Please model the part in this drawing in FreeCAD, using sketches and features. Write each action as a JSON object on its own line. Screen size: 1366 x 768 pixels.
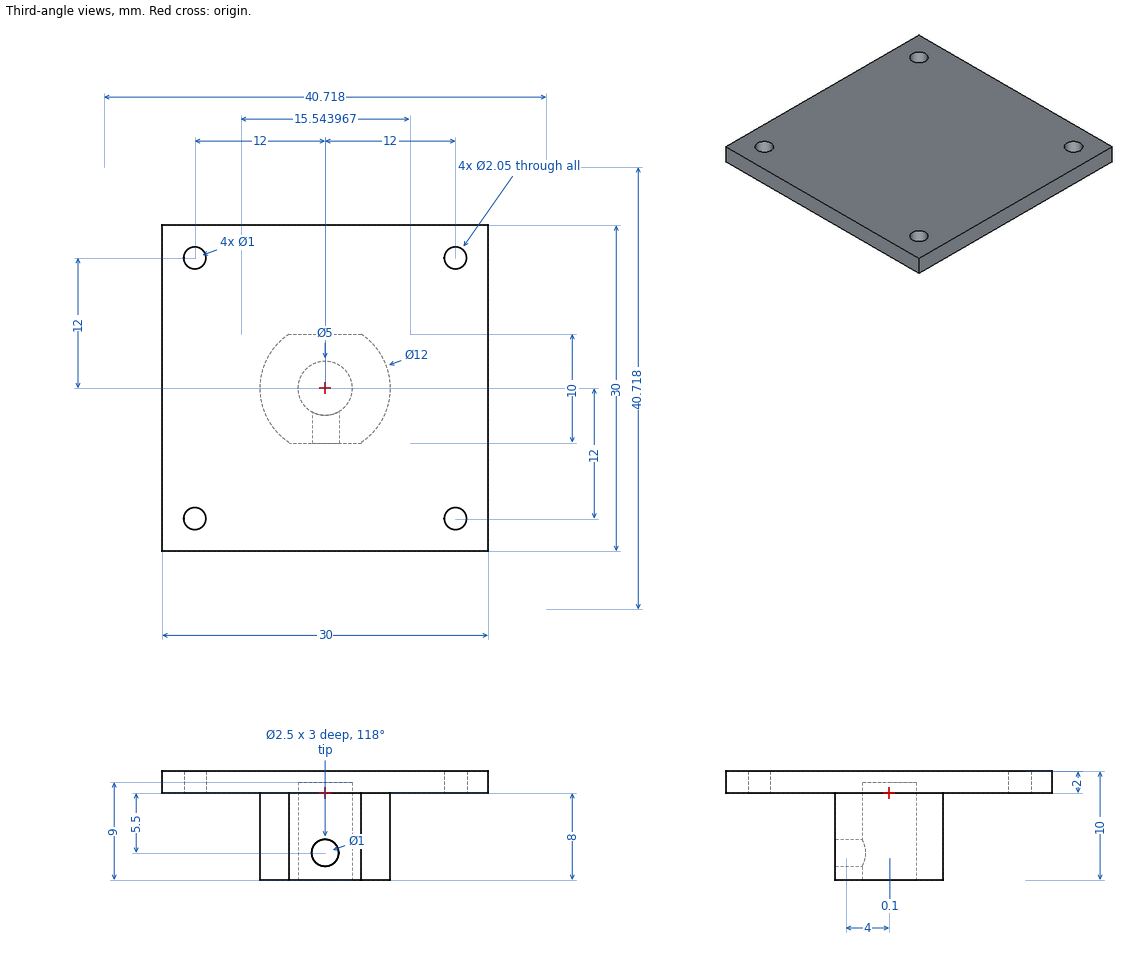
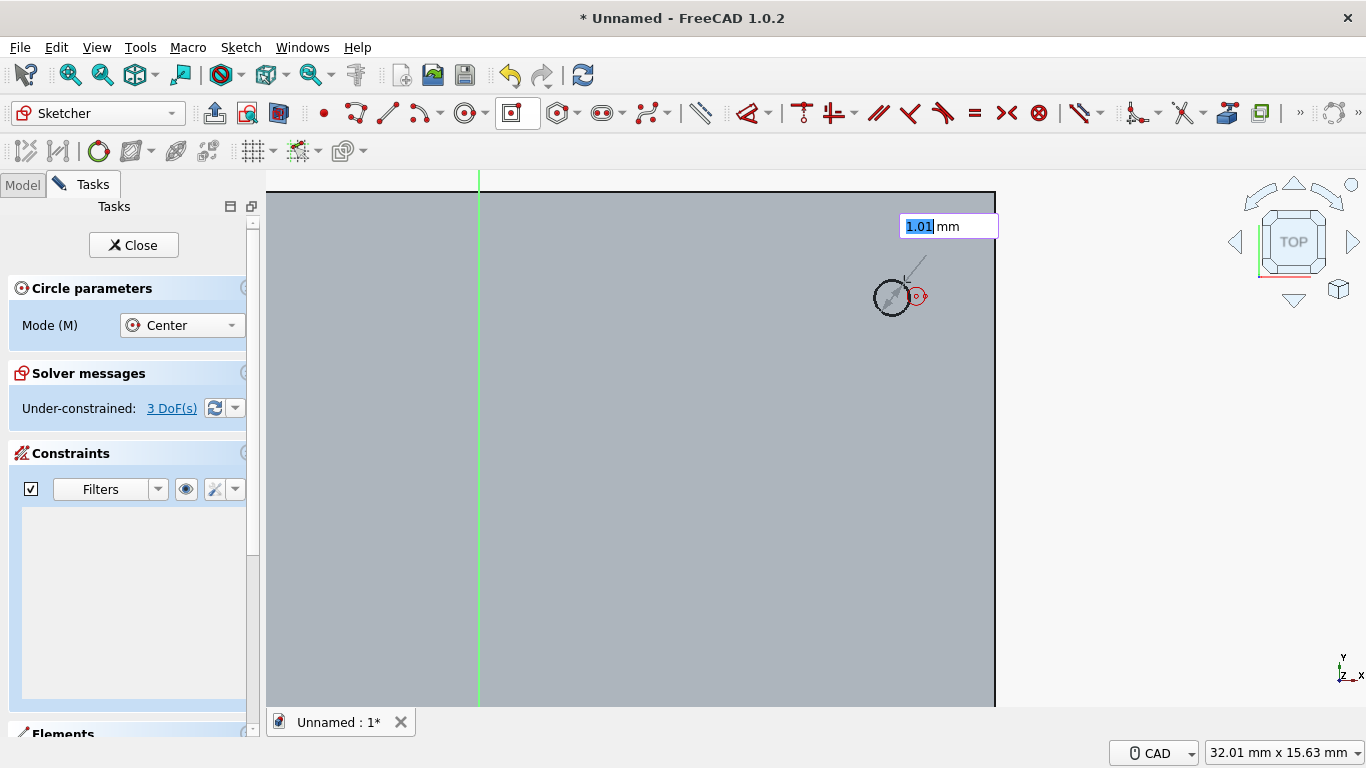
{"action": "left_click", "coordinate": [904, 282]}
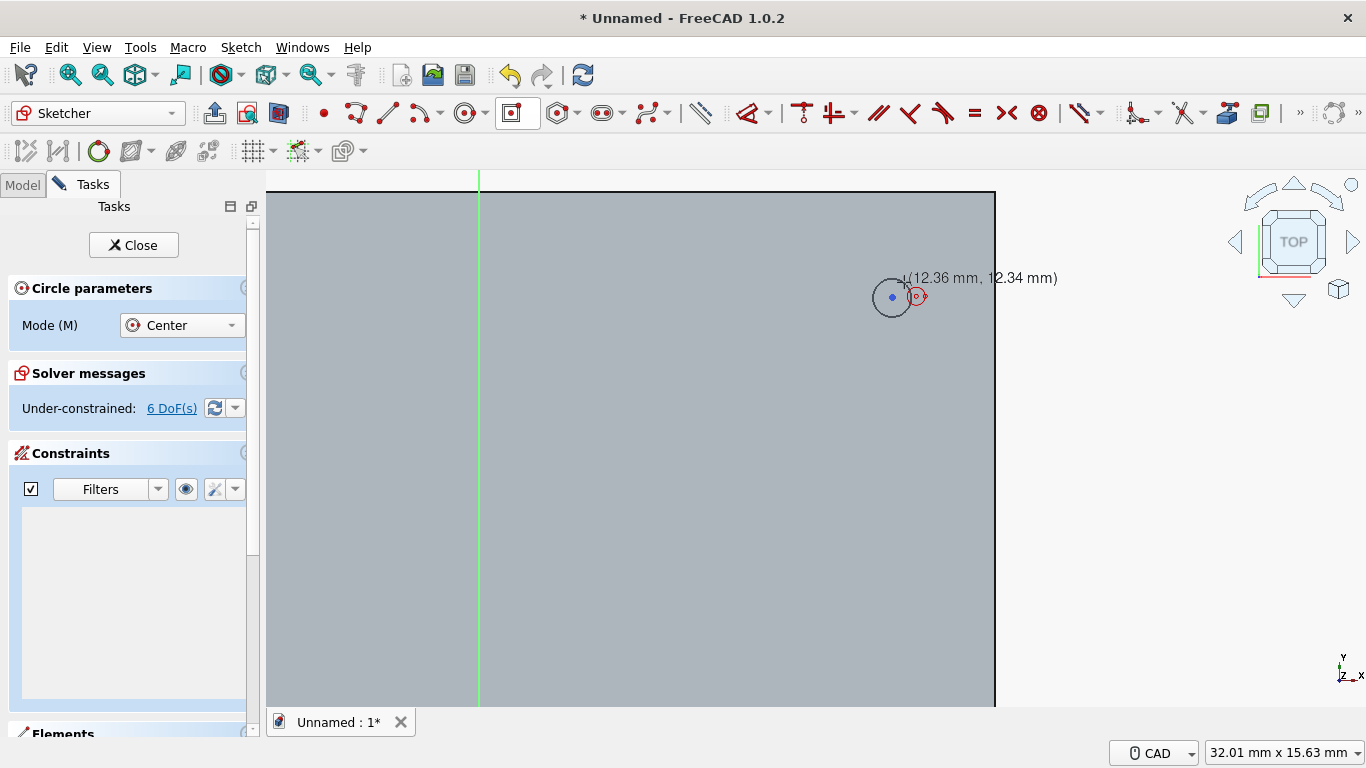
{"action": "scroll", "coordinate": [904, 282], "scroll_direction": "down", "scroll_amount": 5}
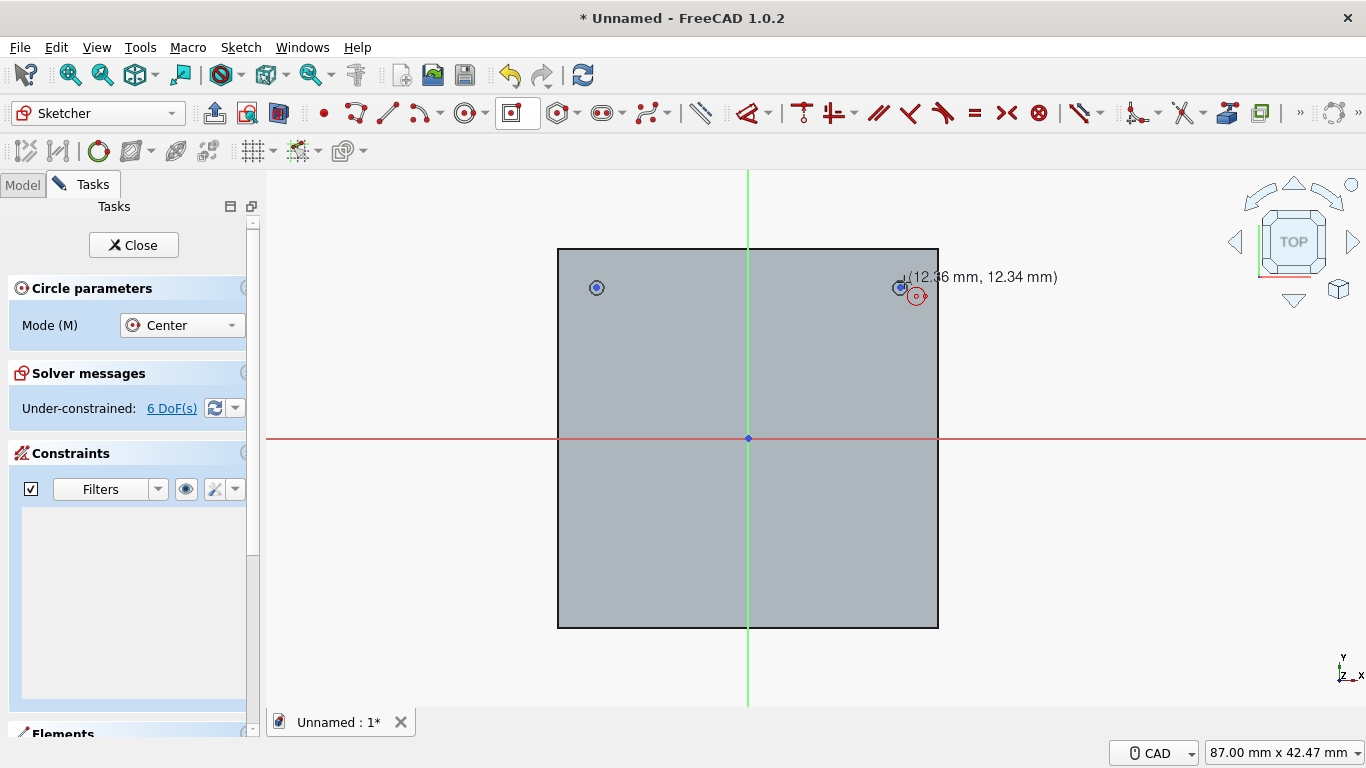
{"action": "scroll", "coordinate": [900, 590], "scroll_direction": "up", "scroll_amount": 7}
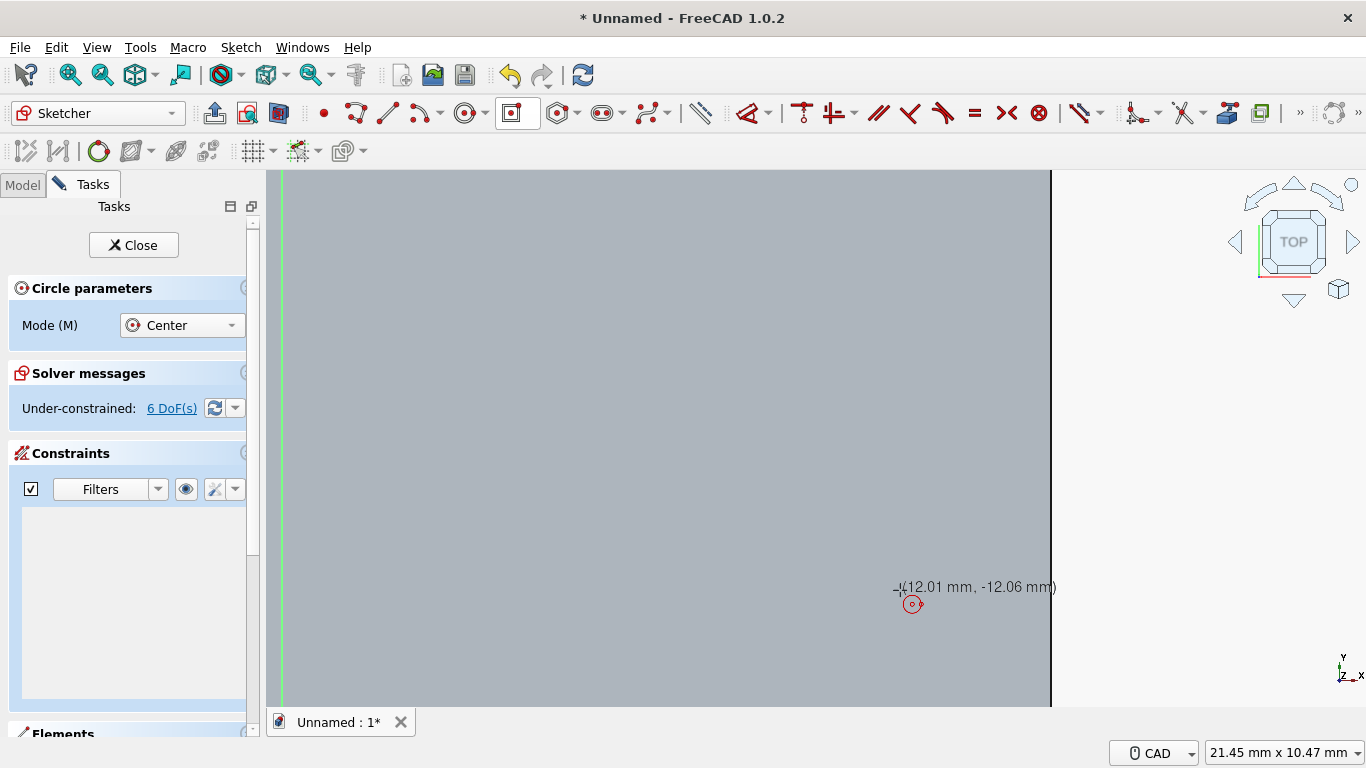
{"action": "scroll", "coordinate": [900, 591], "scroll_direction": "down", "scroll_amount": 7}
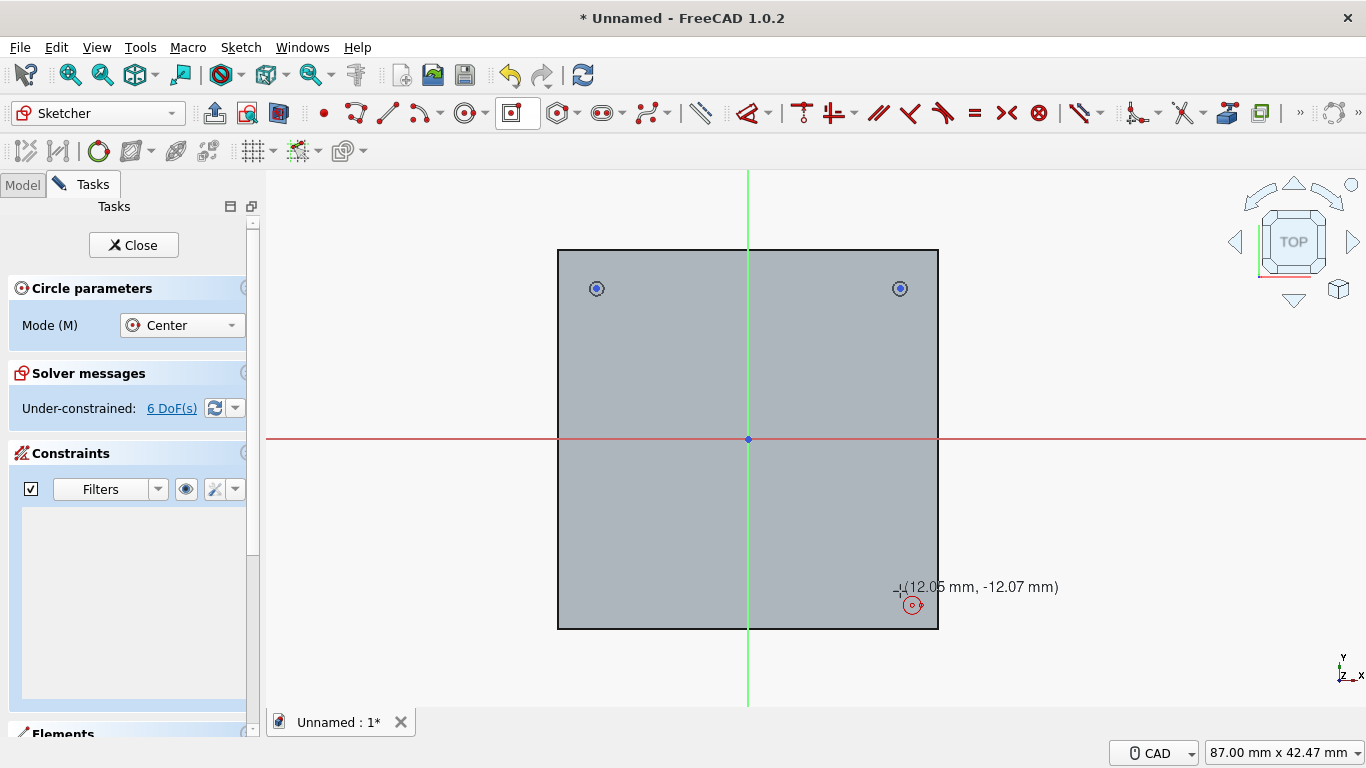
{"action": "left_click", "coordinate": [900, 591]}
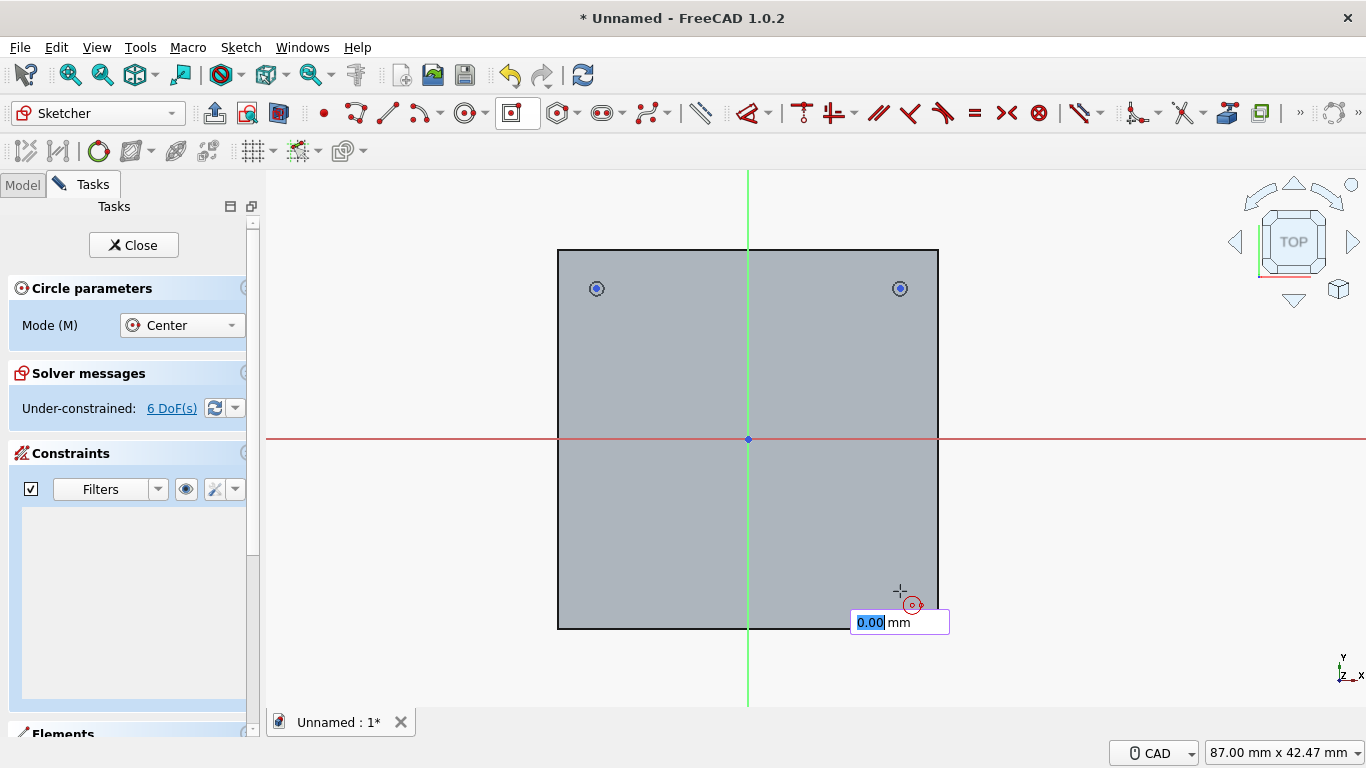
{"action": "scroll", "coordinate": [904, 587], "scroll_direction": "up", "scroll_amount": 5}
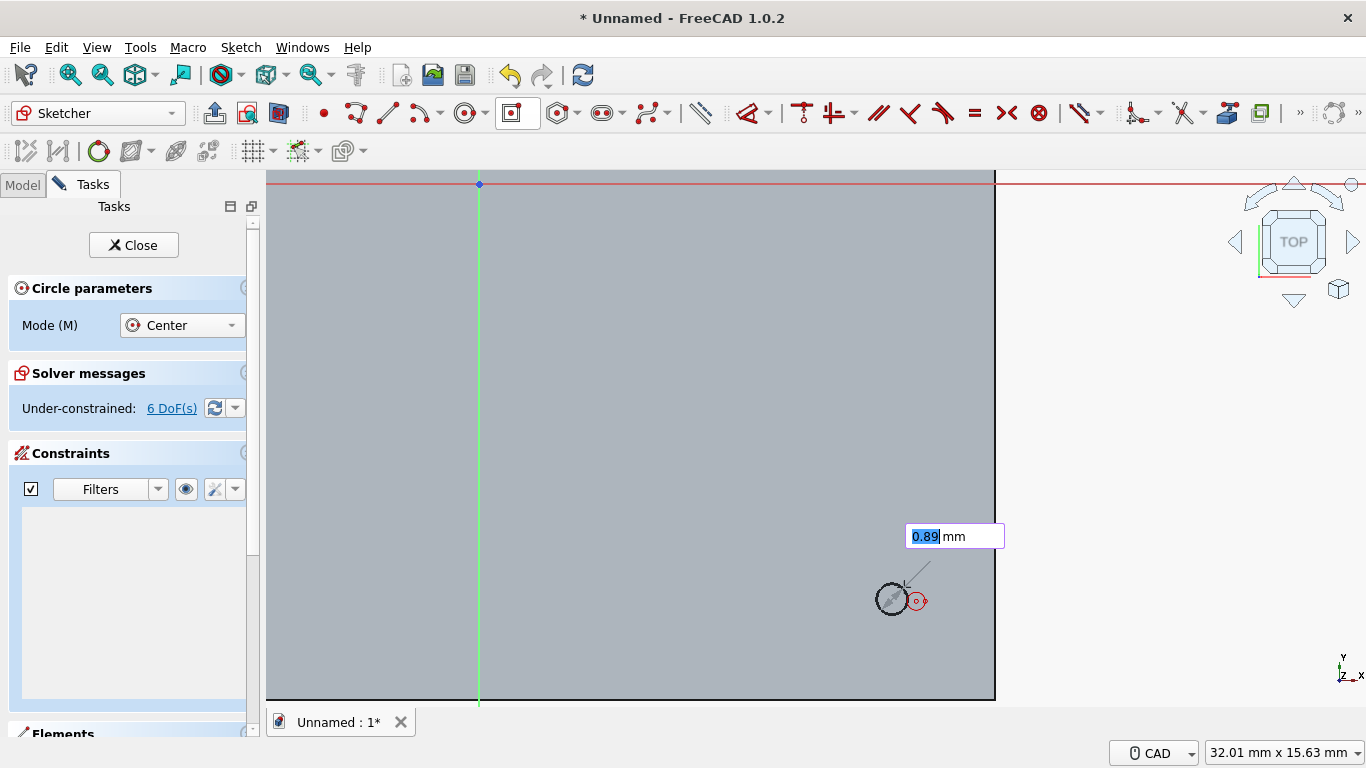
{"action": "left_click", "coordinate": [904, 584]}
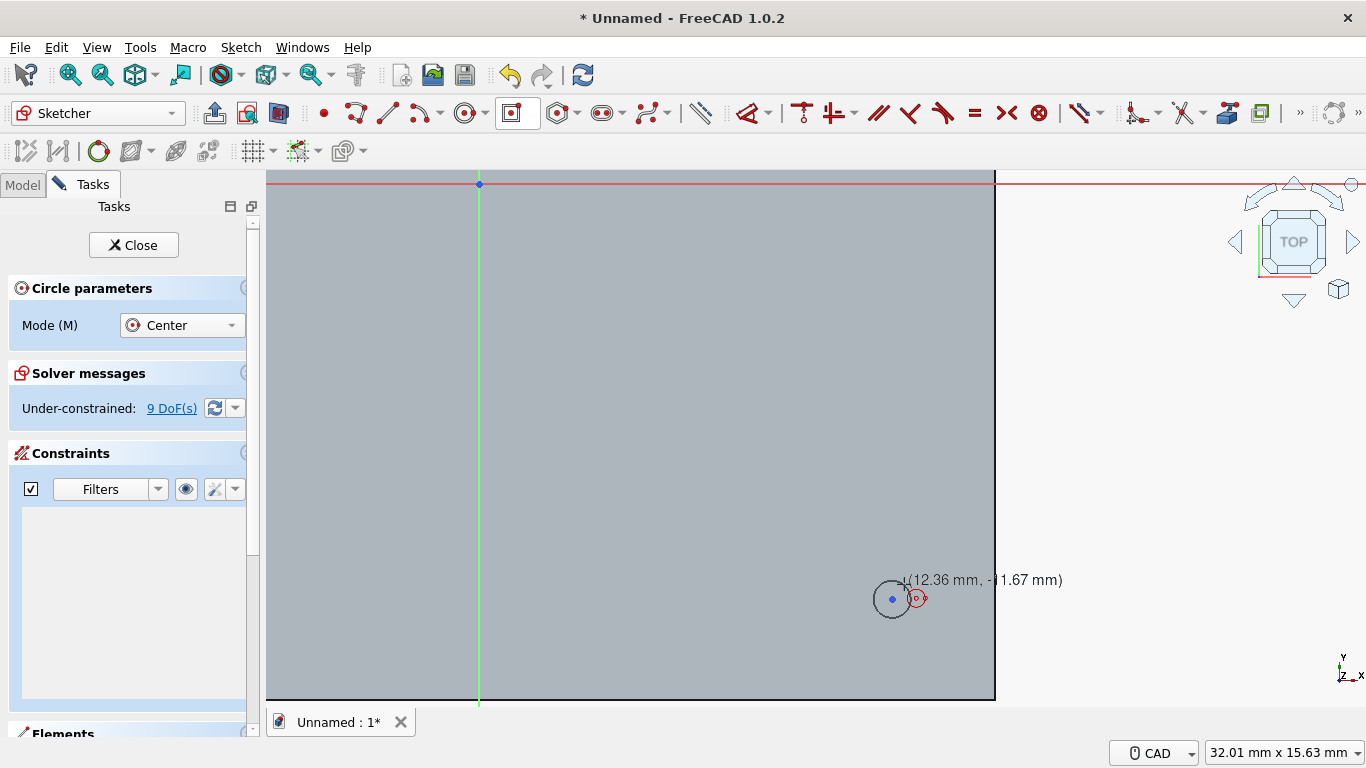
{"action": "scroll", "coordinate": [904, 587], "scroll_direction": "down", "scroll_amount": 5}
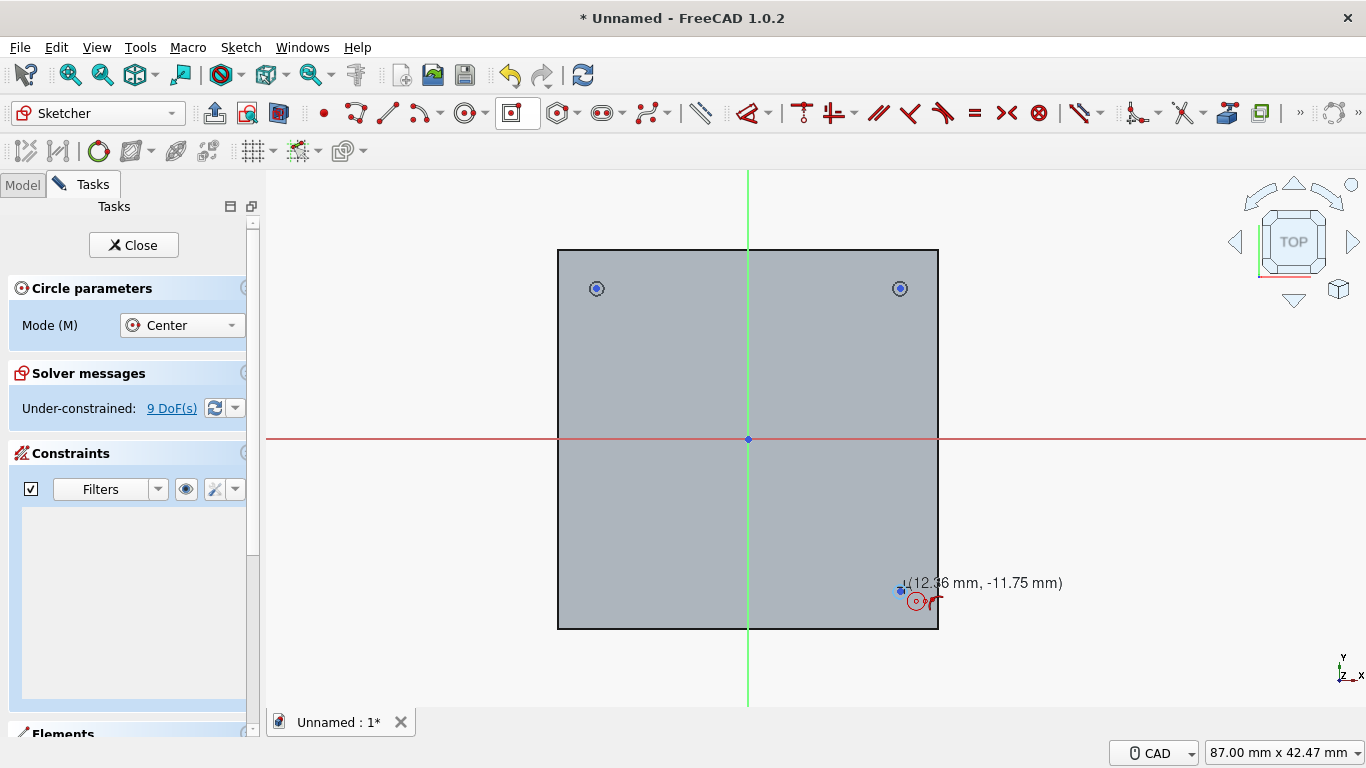
{"action": "scroll", "coordinate": [596, 591], "scroll_direction": "up", "scroll_amount": 7}